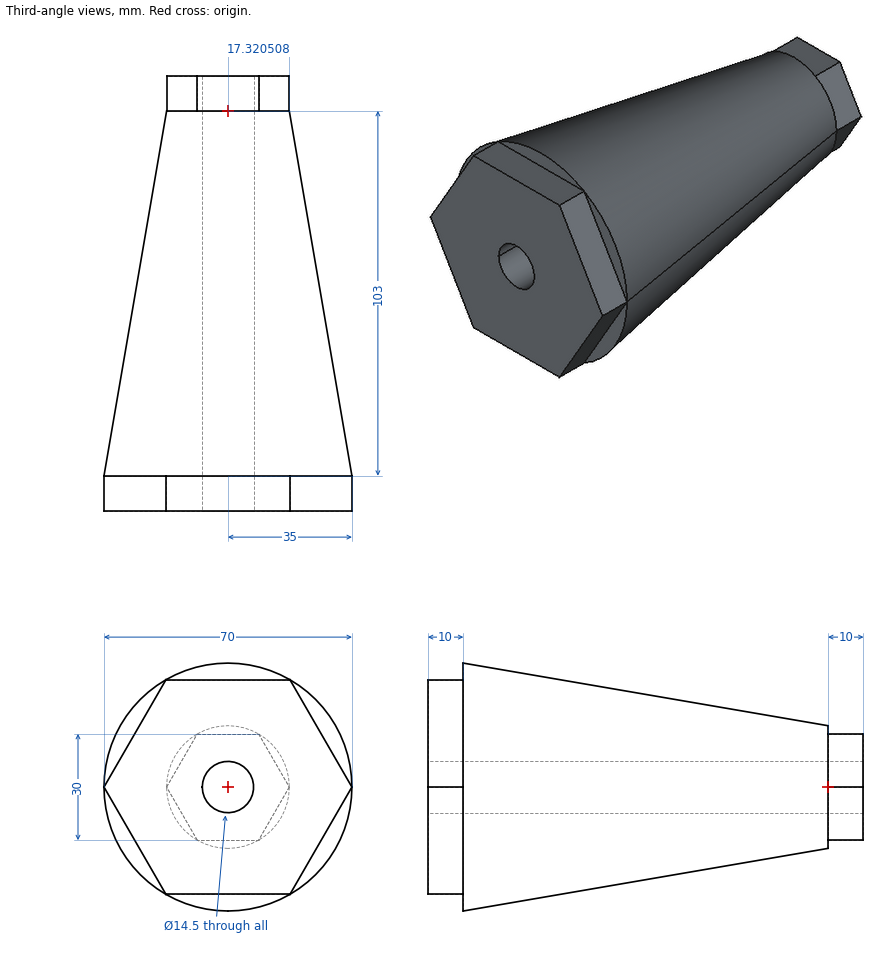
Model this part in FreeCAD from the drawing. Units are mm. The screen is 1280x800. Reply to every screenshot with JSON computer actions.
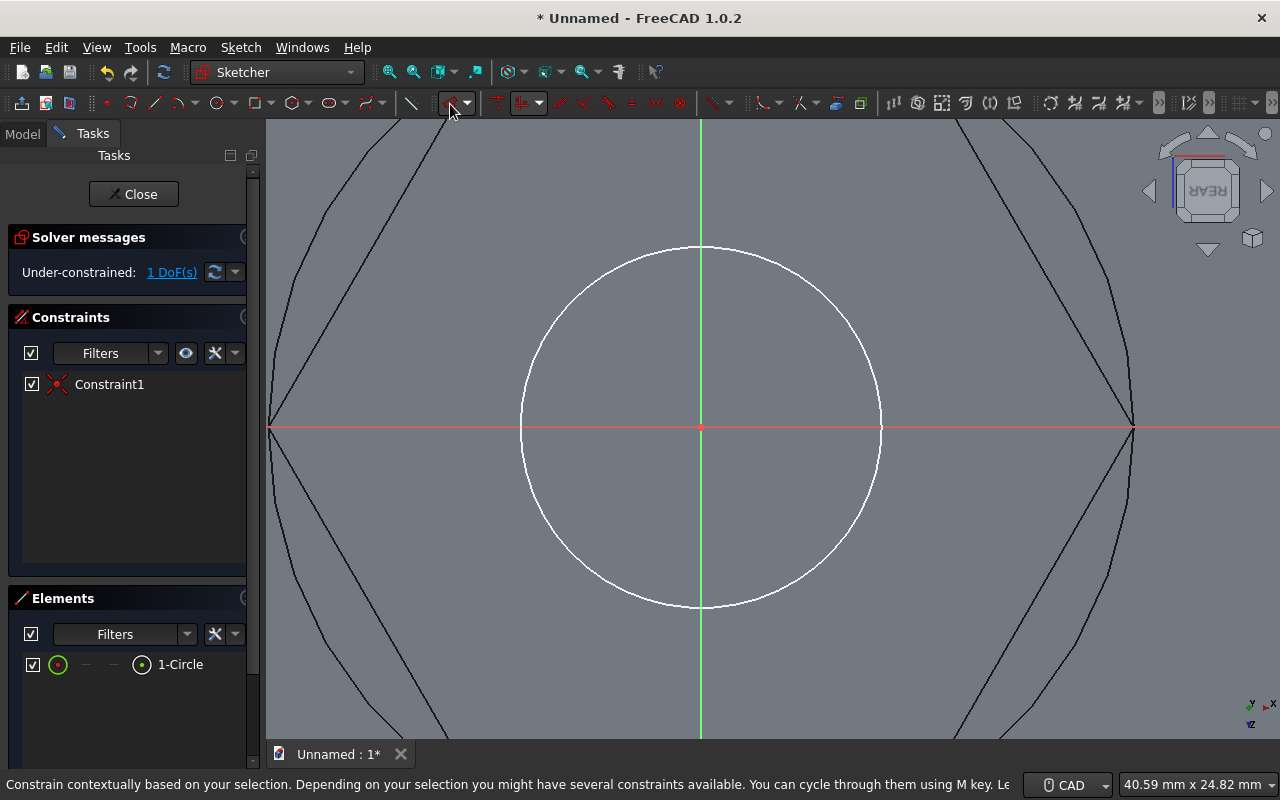
{"action": "left_click", "coordinate": [828, 299]}
{"action": "left_click", "coordinate": [850, 276]}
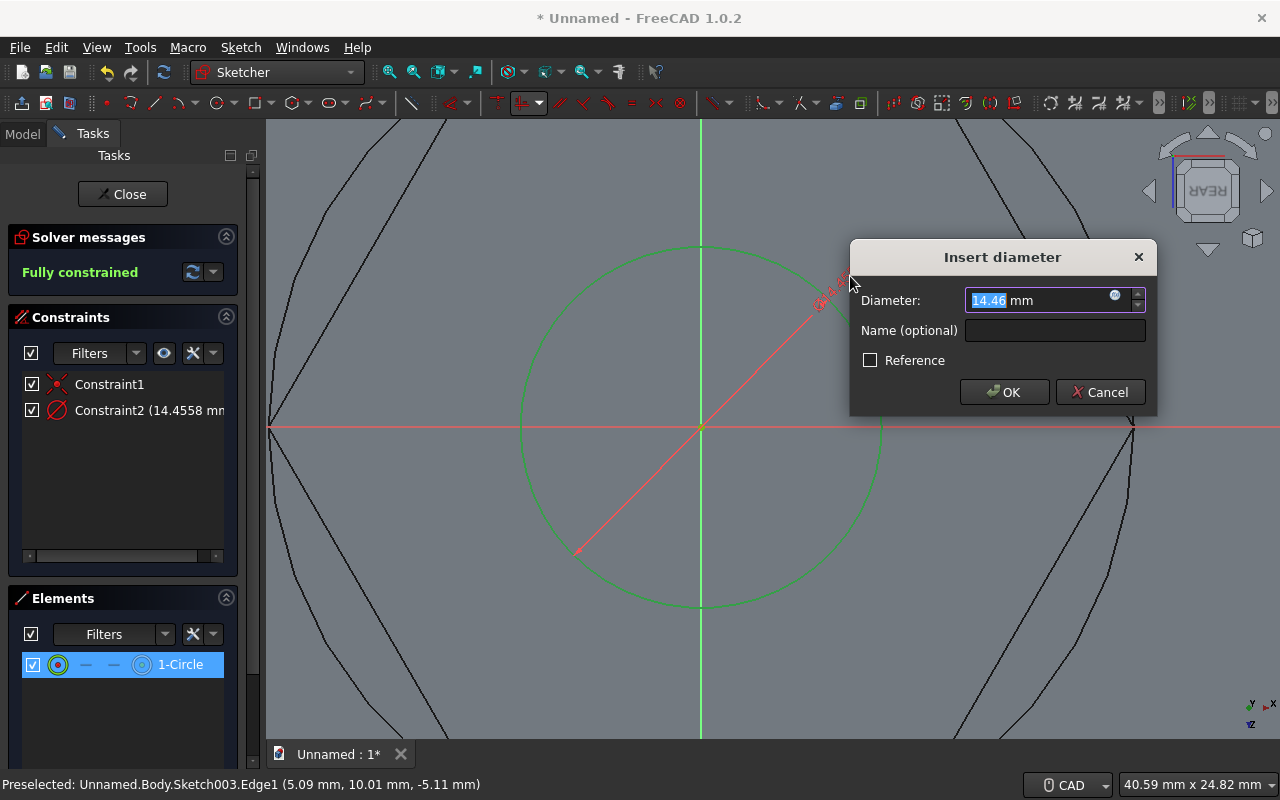
{"action": "type", "text": "14.5"}
{"action": "key", "text": "Return"}
{"action": "key", "text": "Escape"}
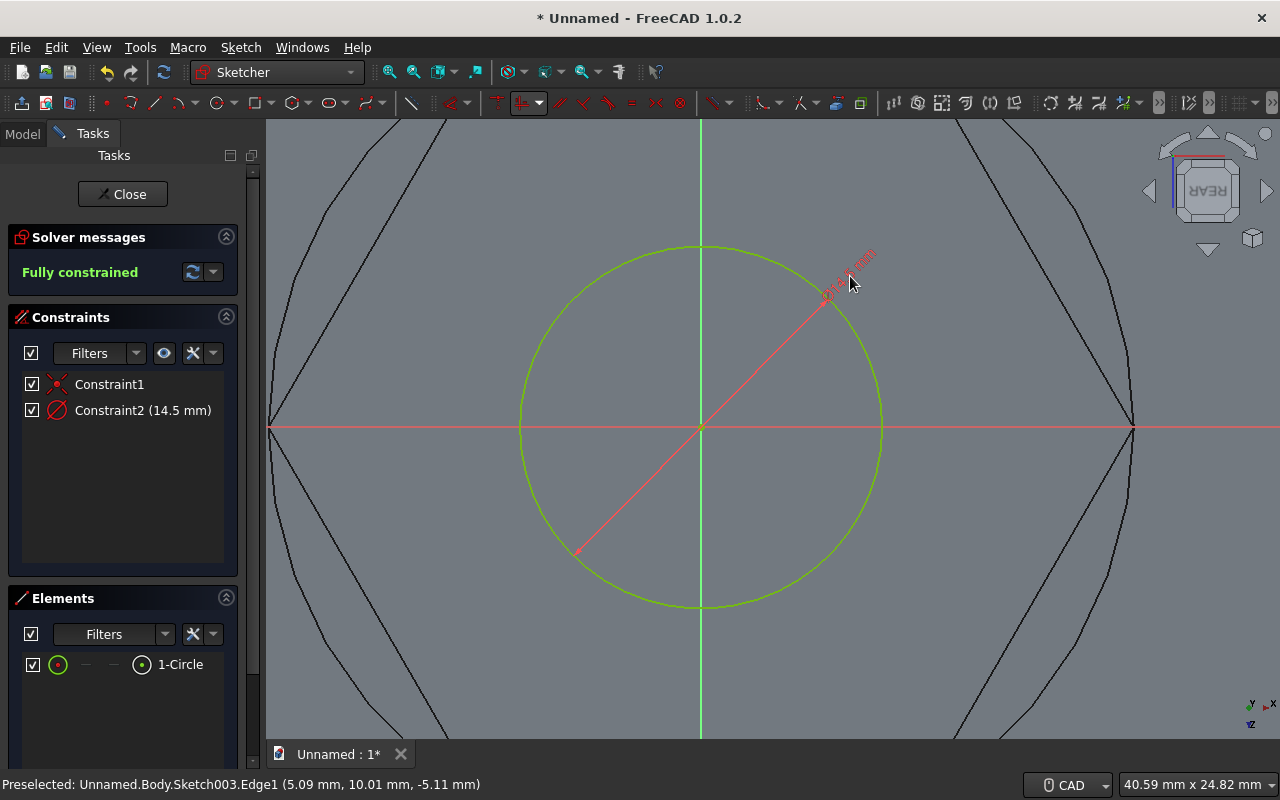
{"action": "left_click", "coordinate": [123, 194]}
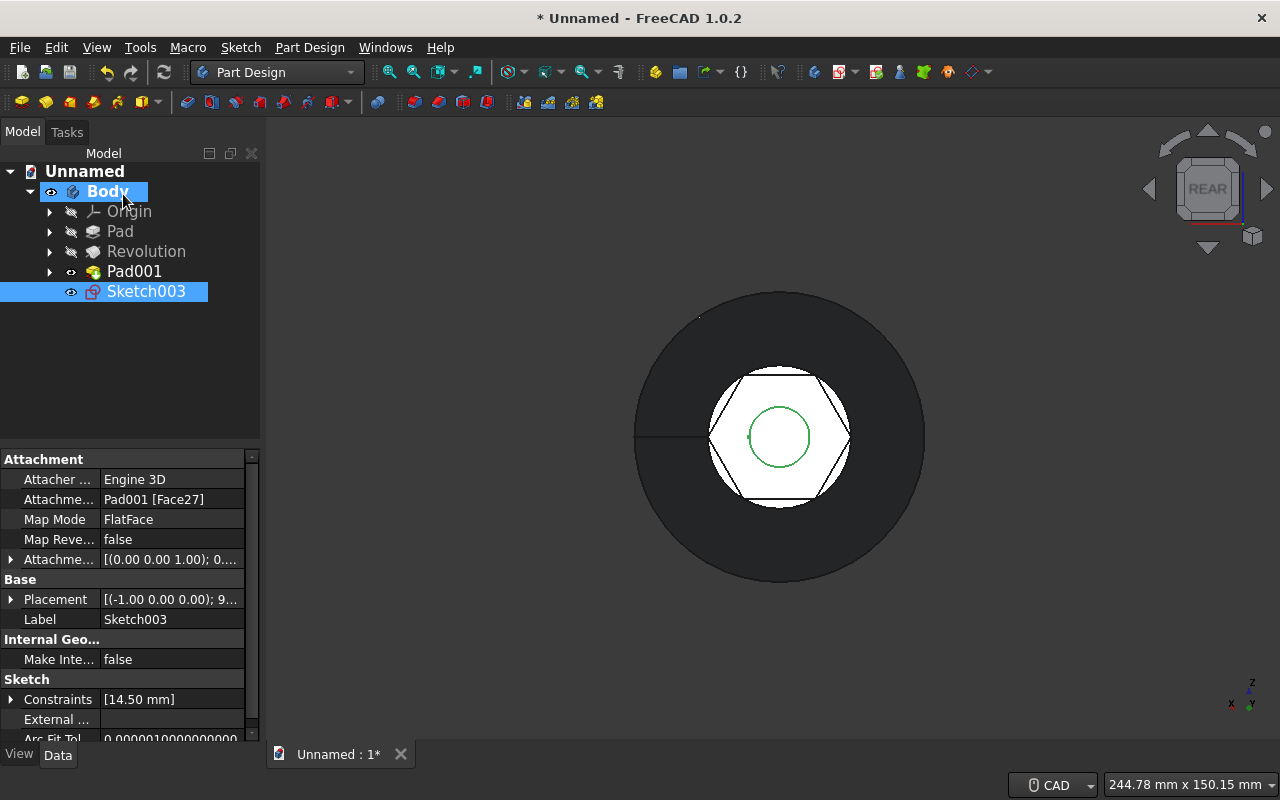
{"action": "left_click", "coordinate": [212, 102]}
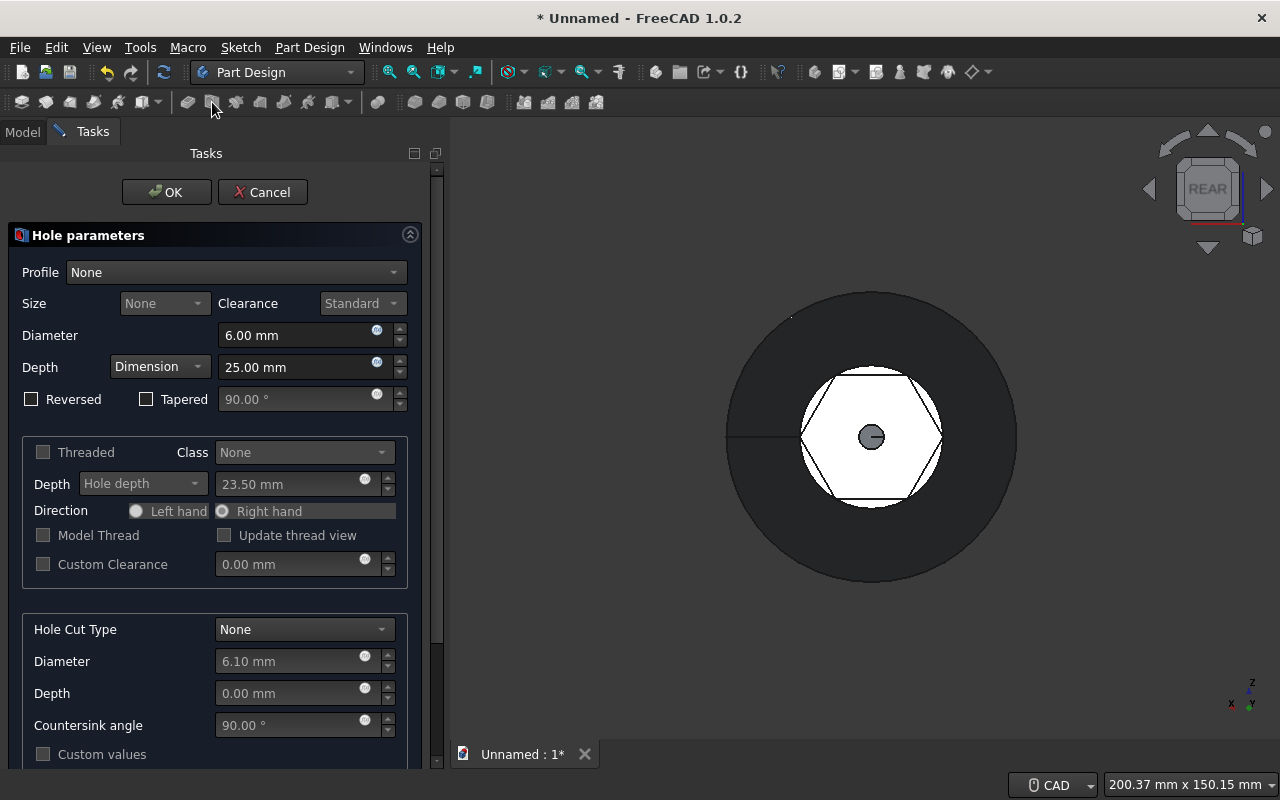
{"action": "triple_click", "coordinate": [305, 335]}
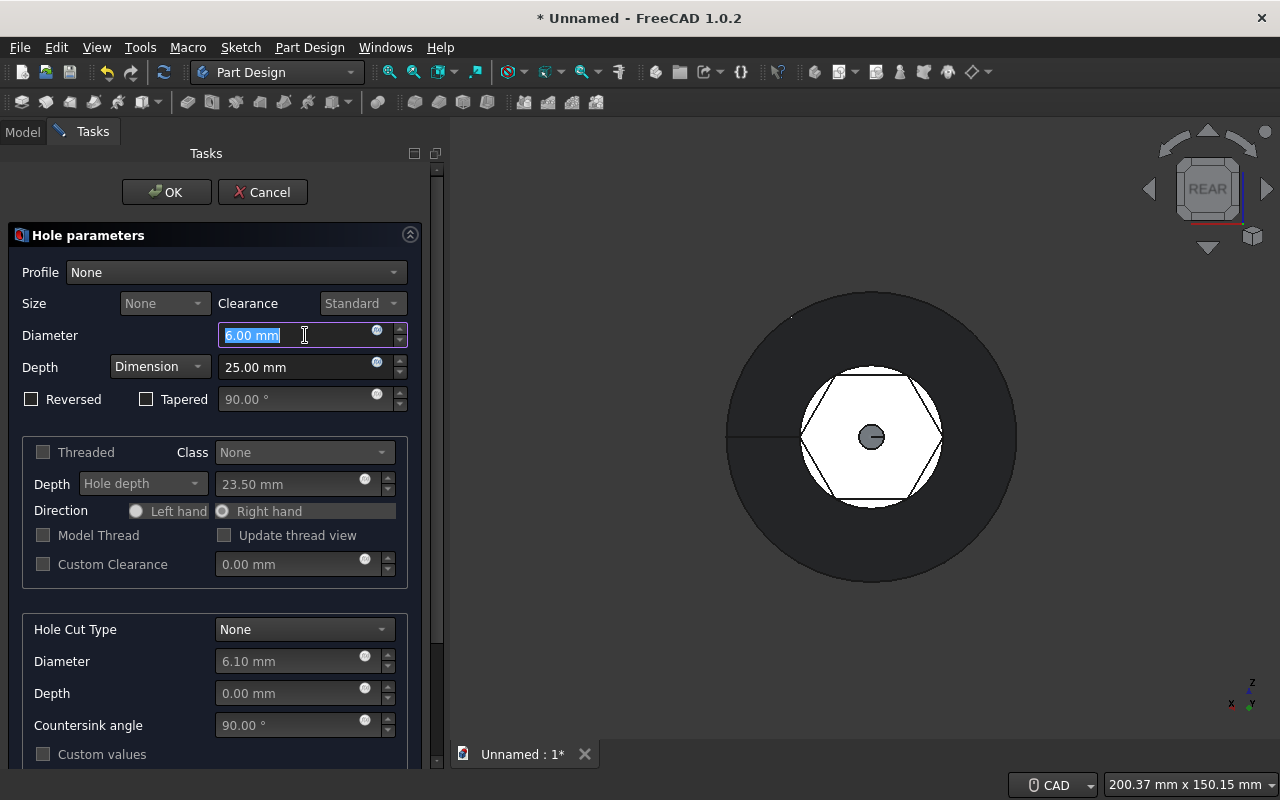
{"action": "type", "text": "14.5"}
{"action": "key", "text": "Tab"}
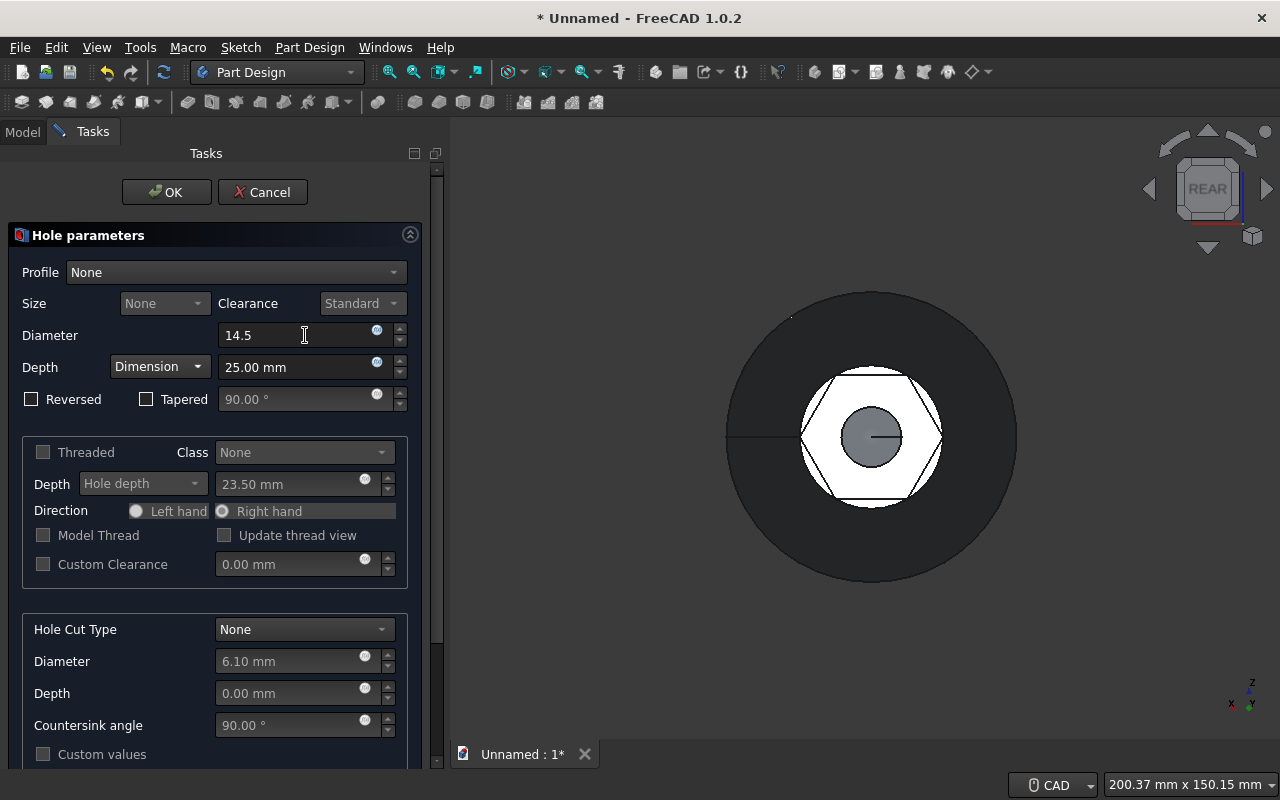
{"action": "left_click", "coordinate": [161, 366]}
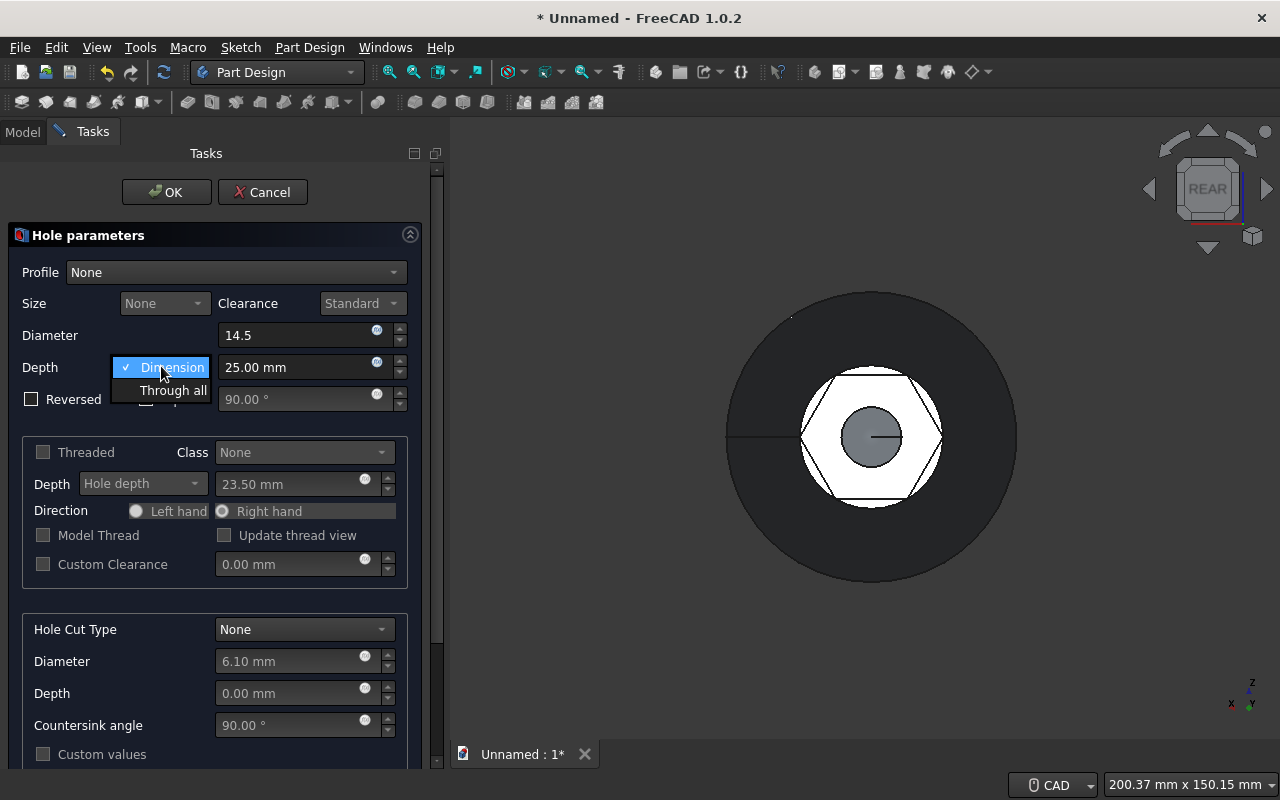
{"action": "left_click", "coordinate": [160, 390]}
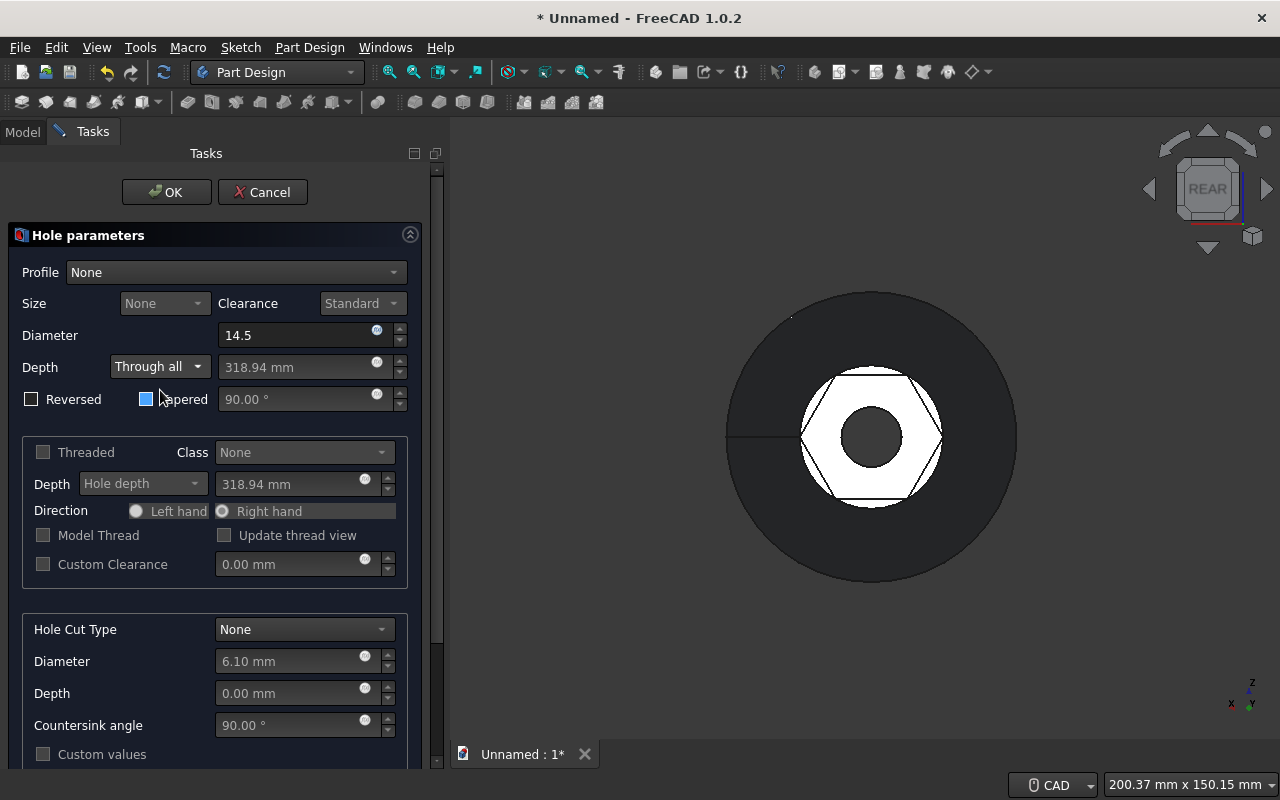
{"action": "left_click", "coordinate": [167, 192]}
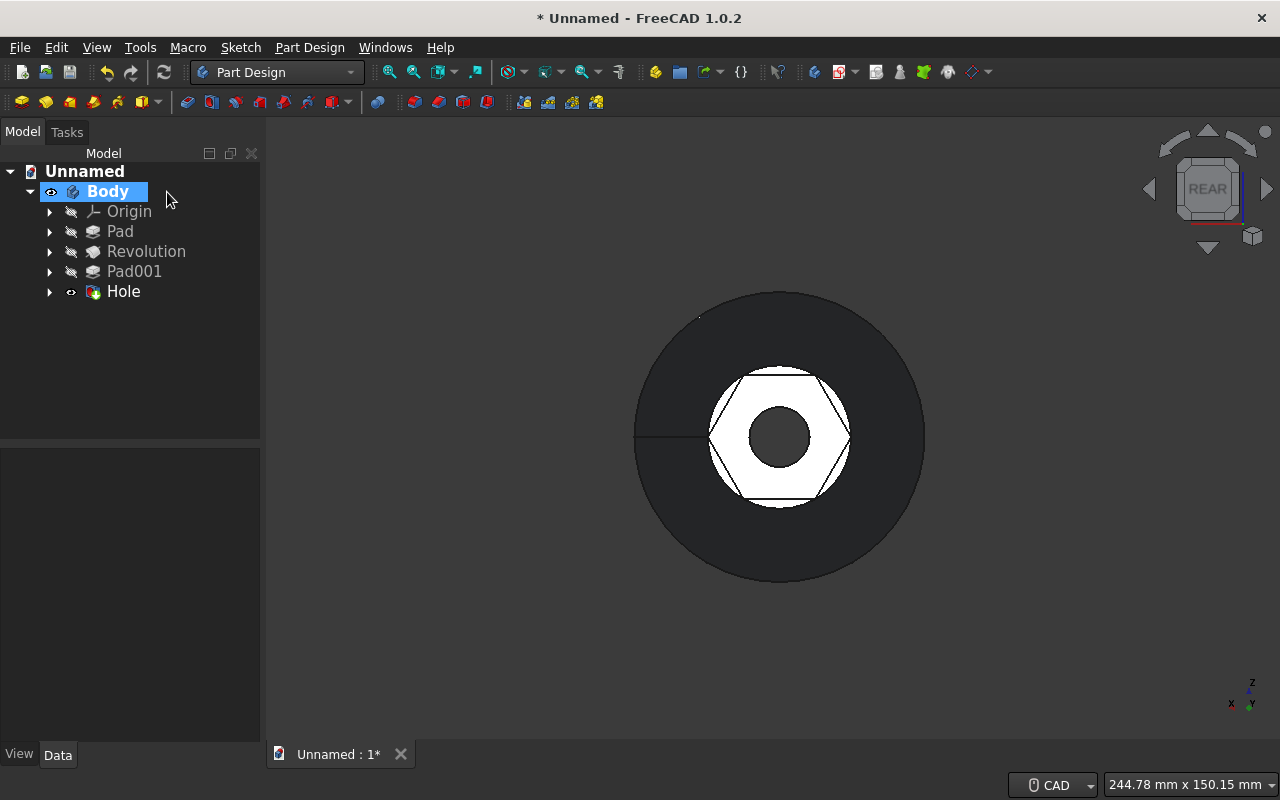
{"action": "key", "text": "0"}